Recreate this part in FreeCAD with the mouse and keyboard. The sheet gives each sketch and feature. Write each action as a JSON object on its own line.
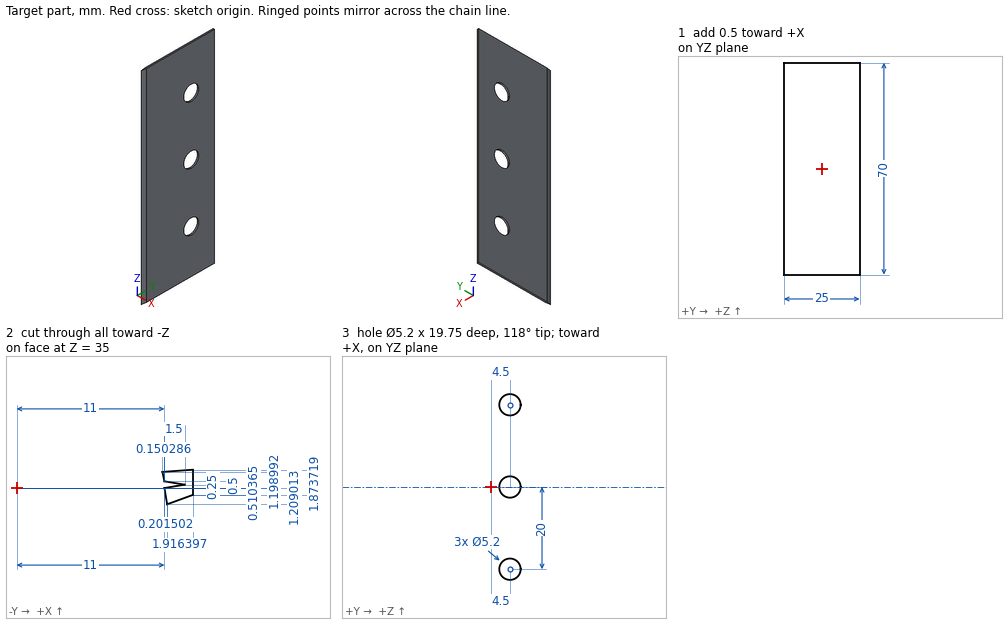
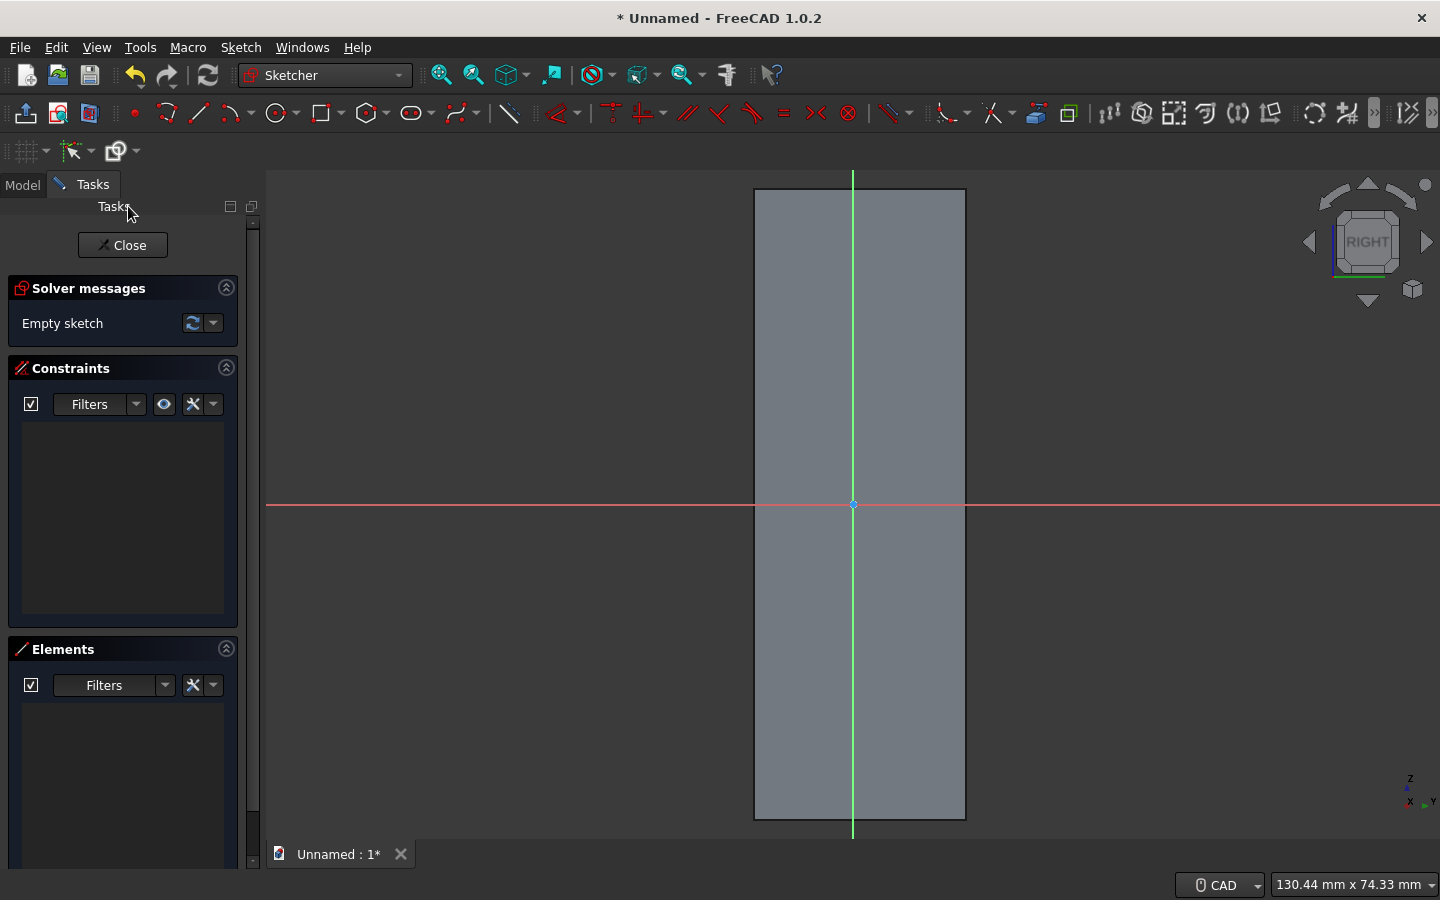
{"action": "left_click", "coordinate": [276, 114]}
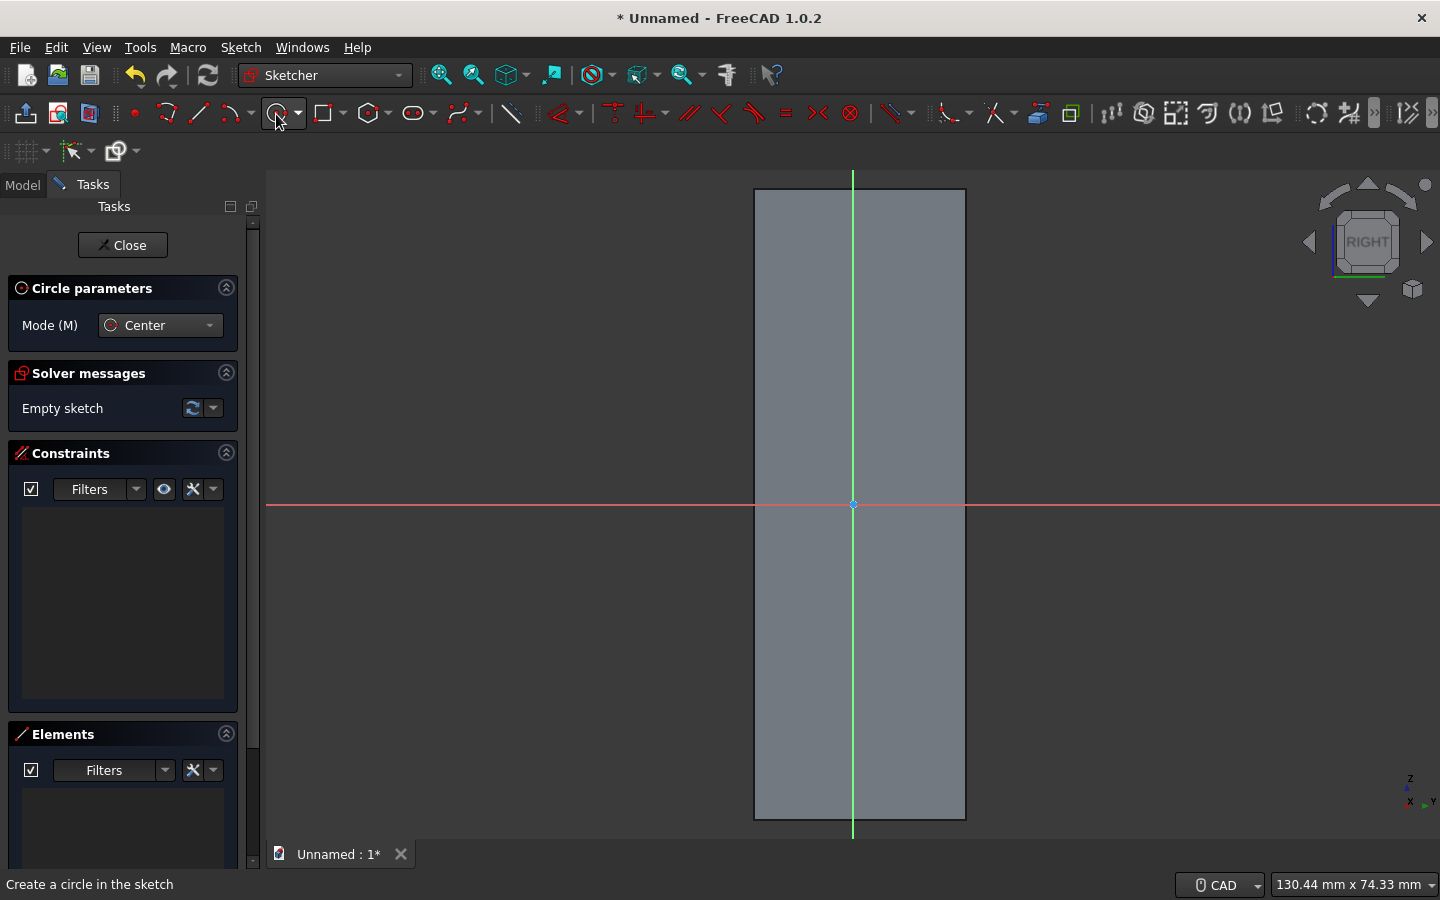
{"action": "left_click", "coordinate": [894, 685]}
{"action": "mouse_move", "coordinate": [910, 668]}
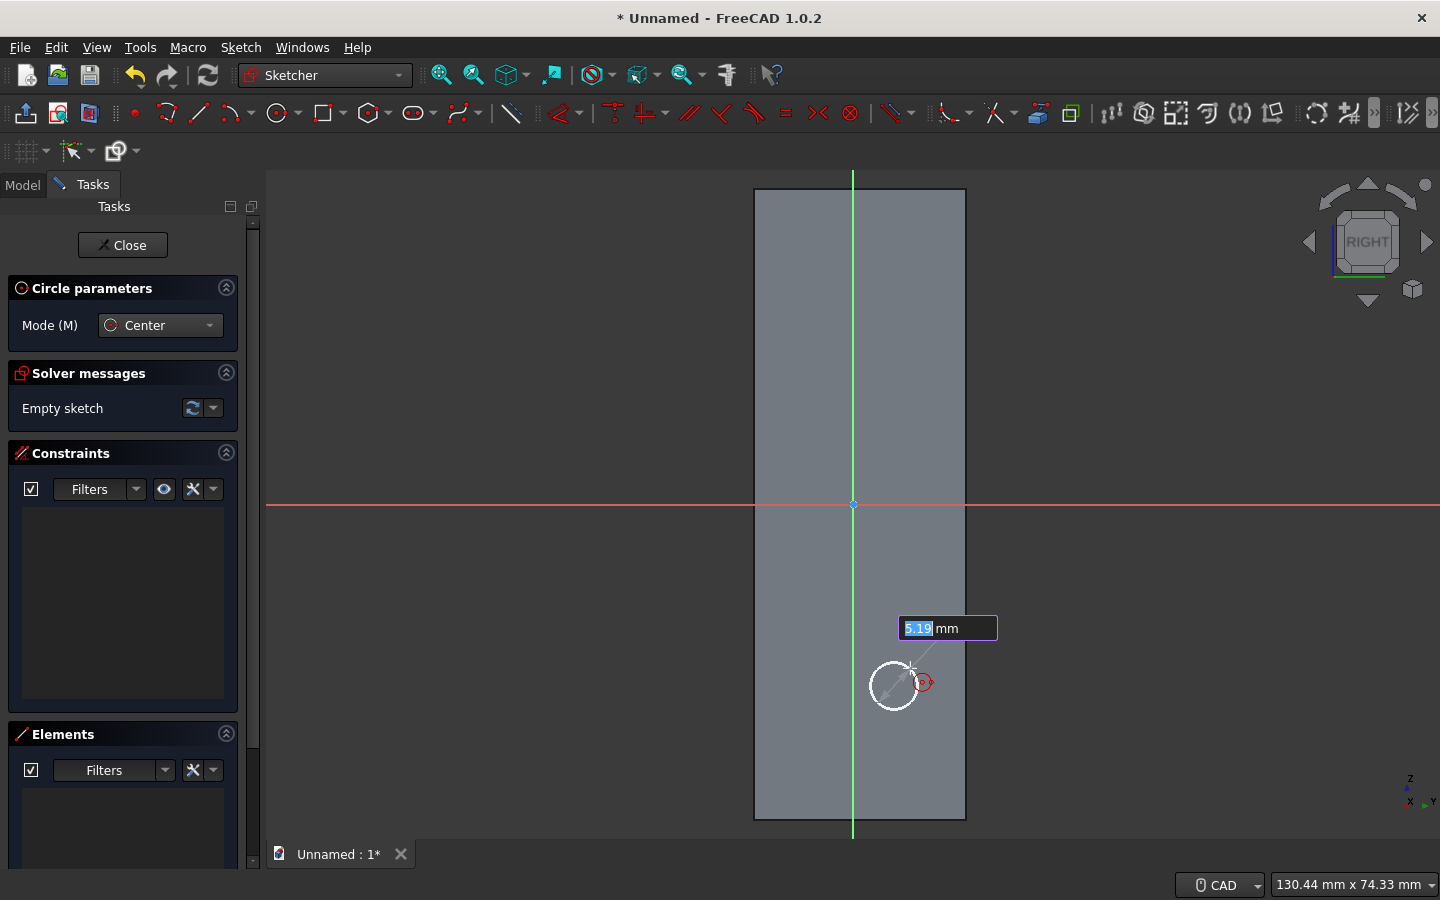
{"action": "type", "text": "5.2"}
{"action": "key", "text": "Return"}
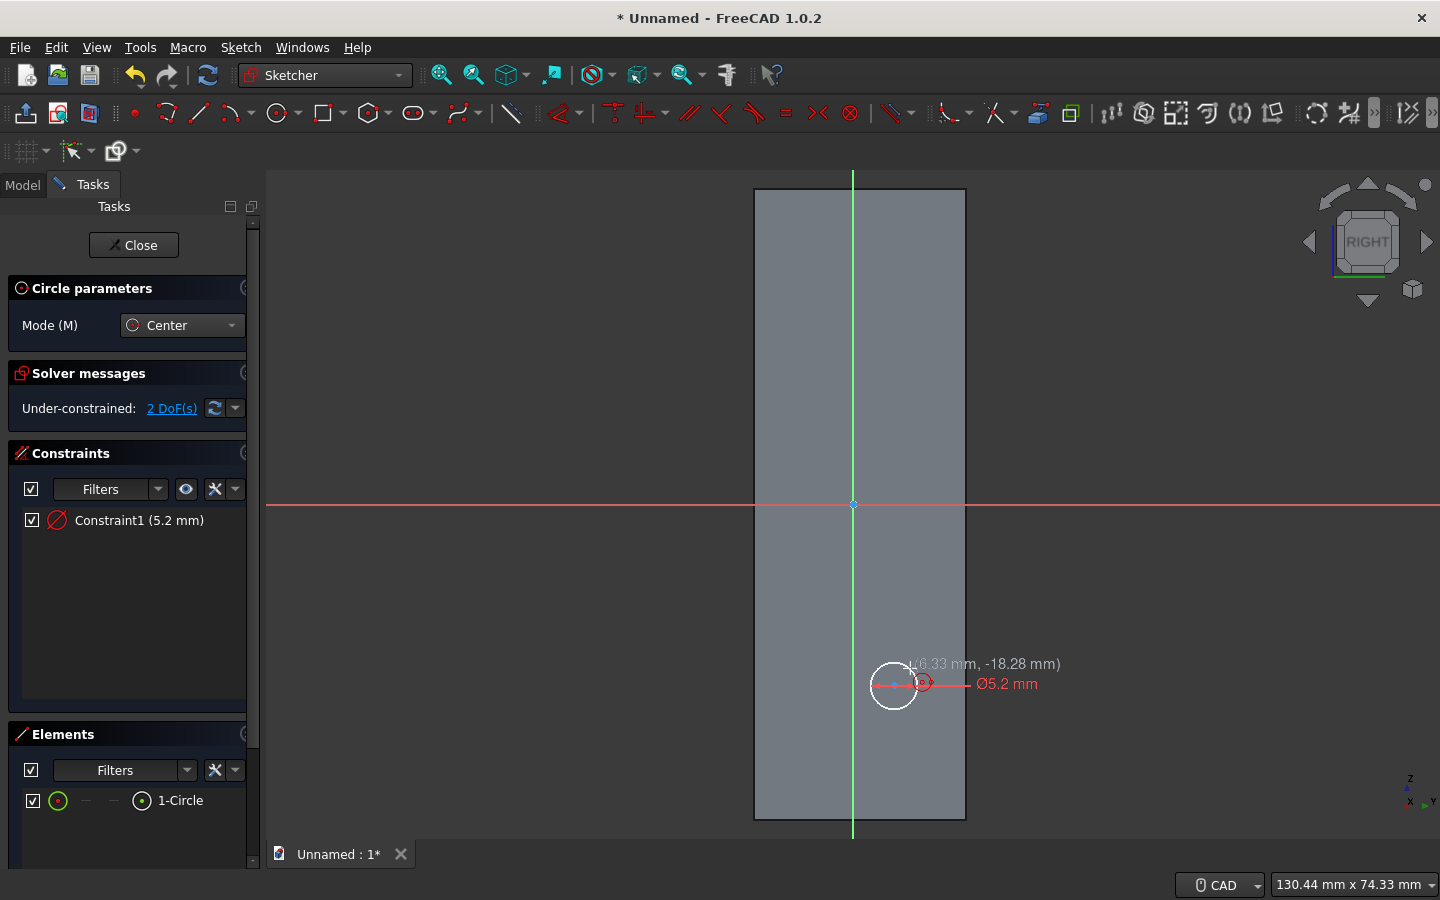
{"action": "left_click", "coordinate": [894, 504]}
{"action": "mouse_move", "coordinate": [910, 488]}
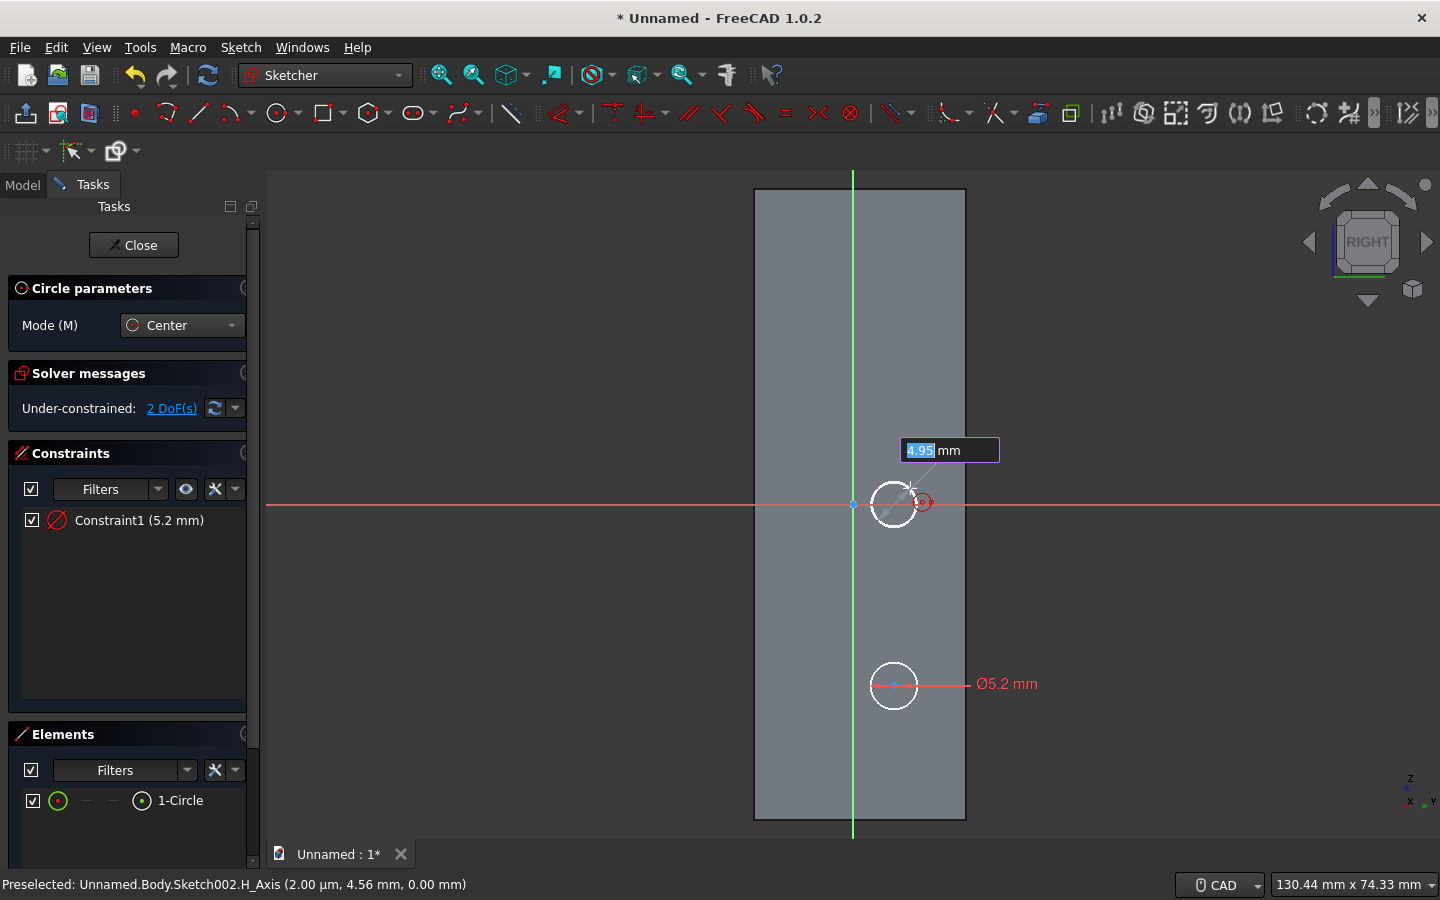
{"action": "type", "text": "5.2"}
{"action": "key", "text": "Return"}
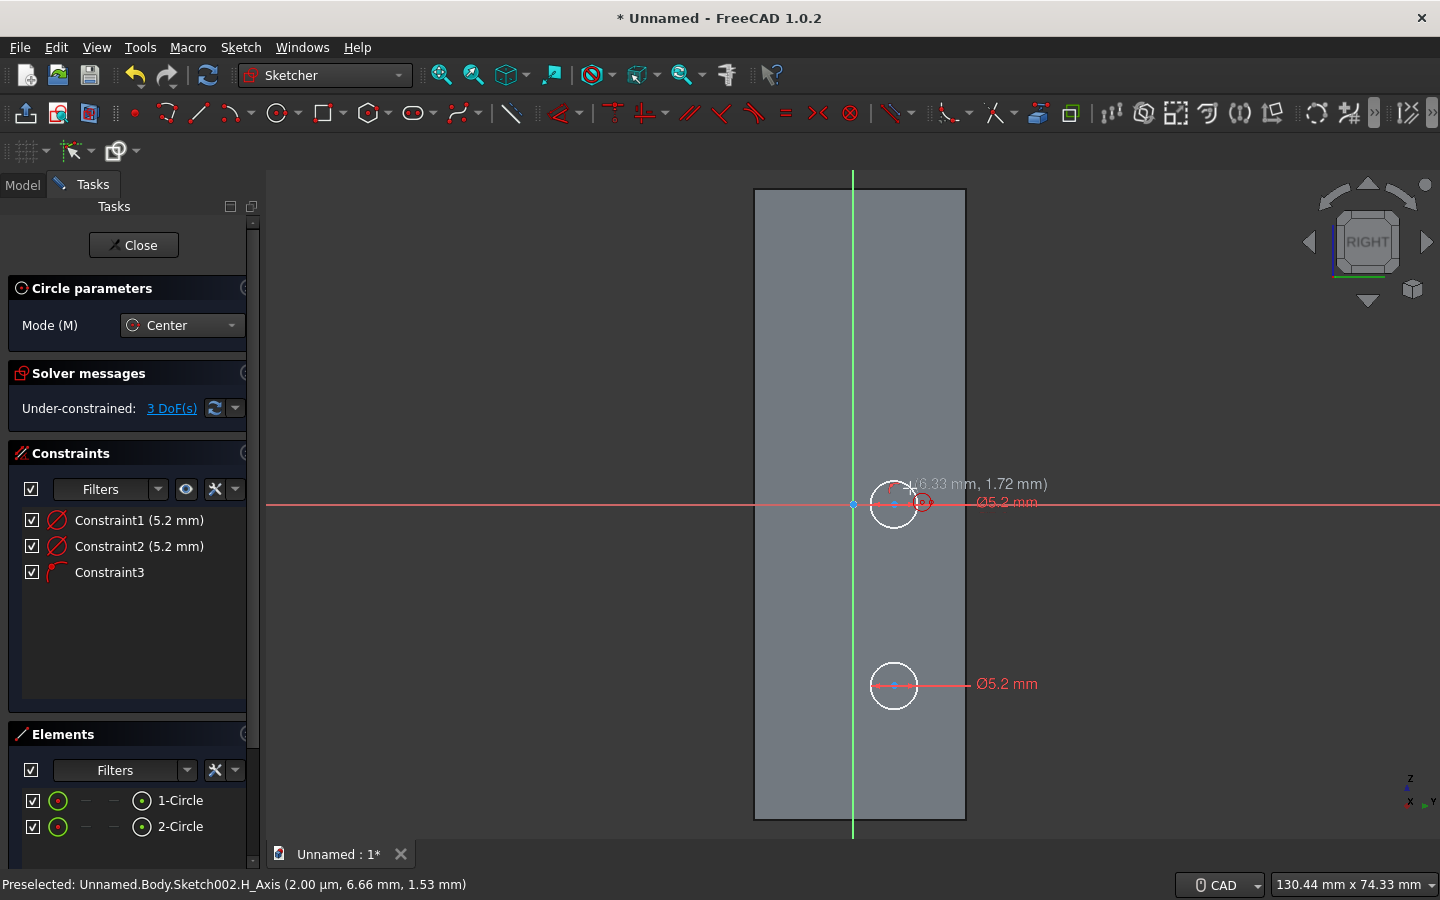
{"action": "left_click", "coordinate": [894, 324]}
{"action": "mouse_move", "coordinate": [910, 308]}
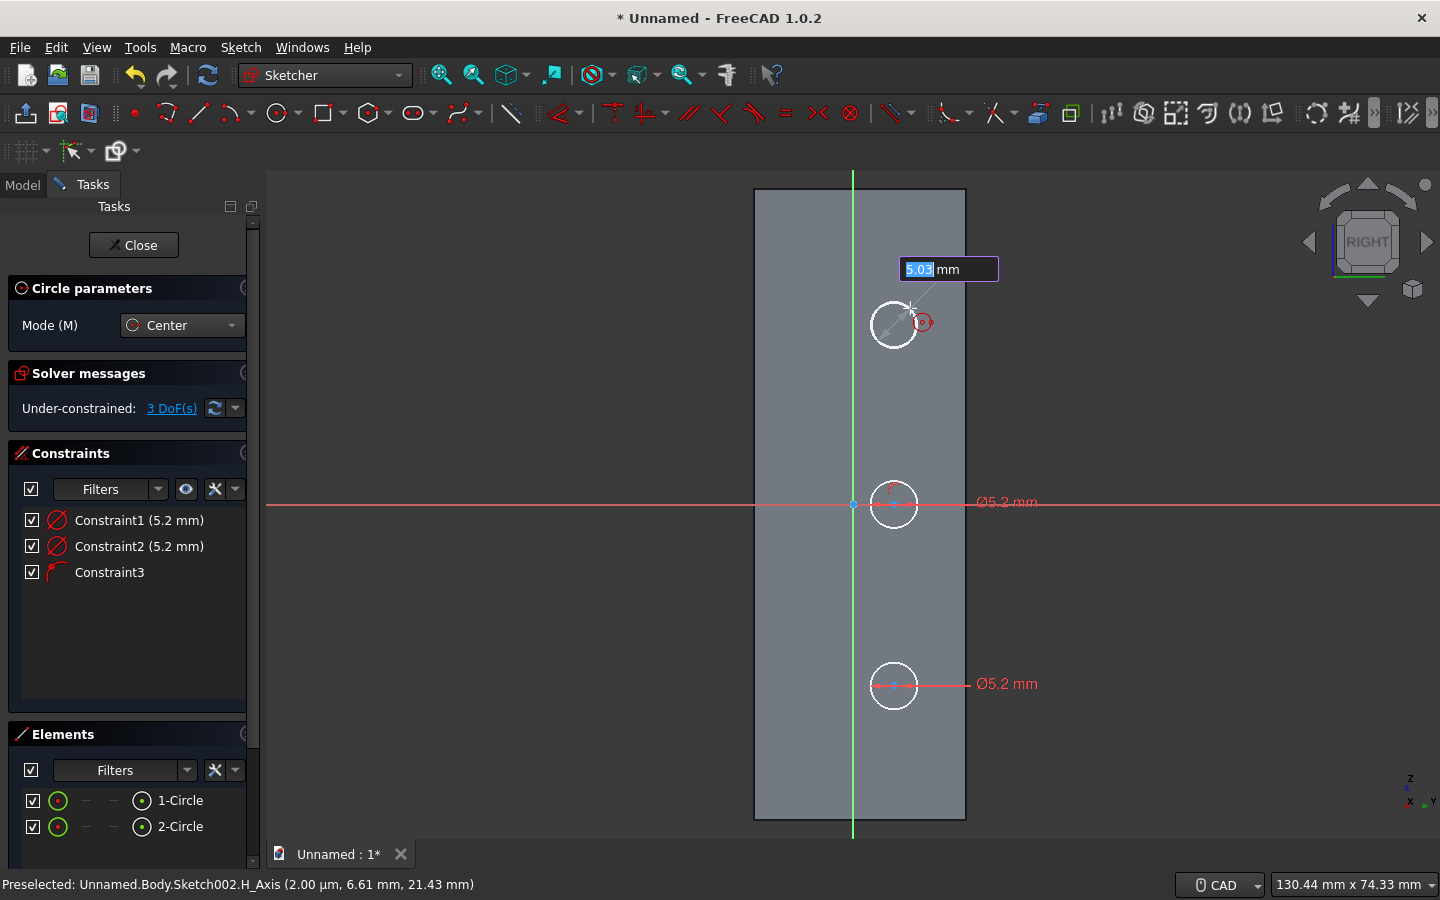
{"action": "type", "text": "5.2"}
{"action": "key", "text": "Return"}
{"action": "key", "text": "Escape"}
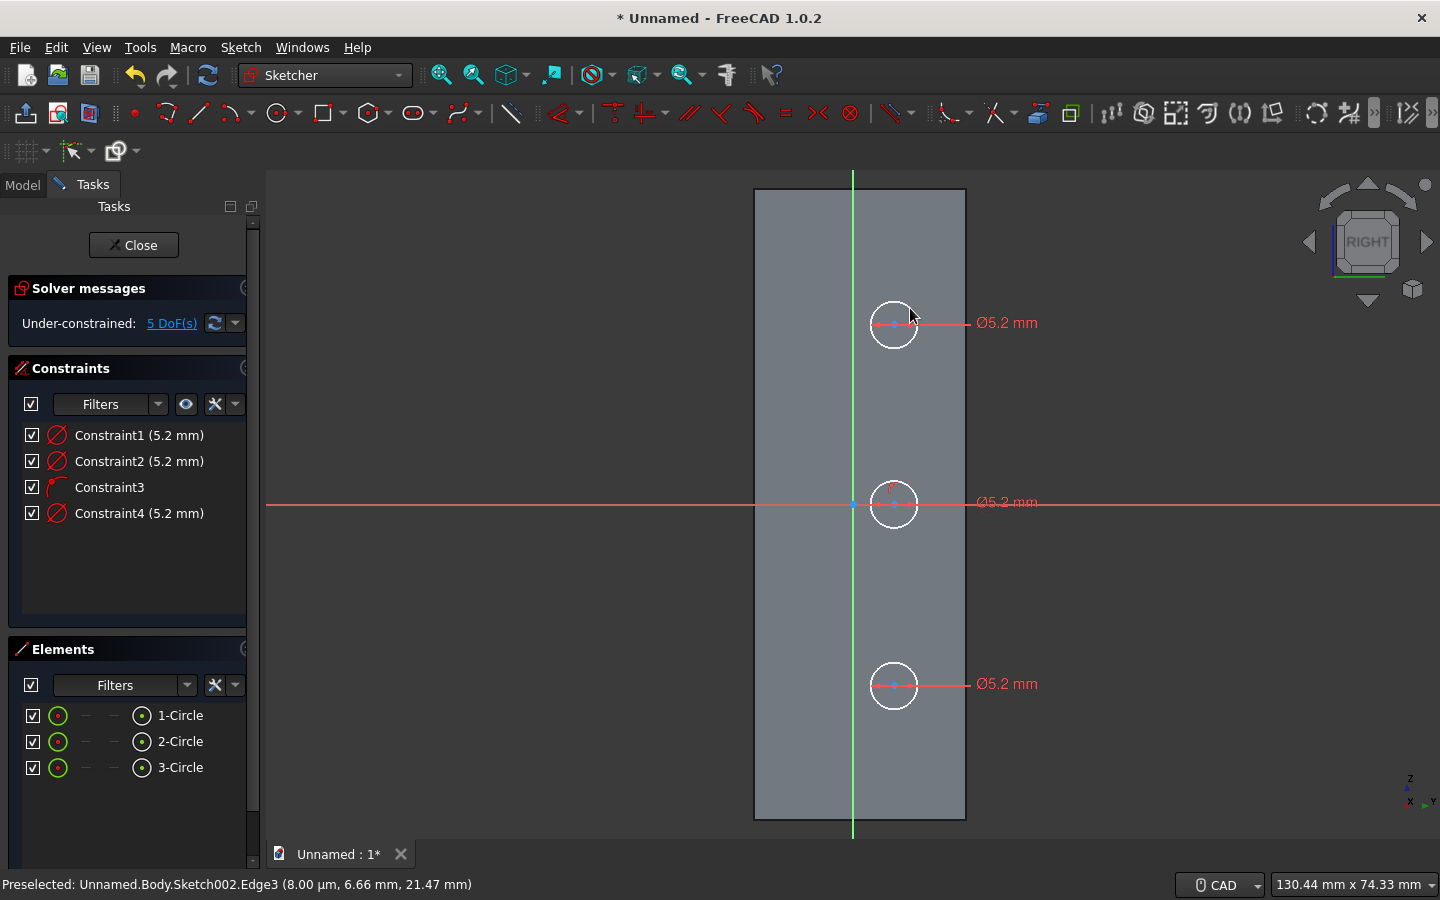
{"action": "left_click", "coordinate": [894, 686]}